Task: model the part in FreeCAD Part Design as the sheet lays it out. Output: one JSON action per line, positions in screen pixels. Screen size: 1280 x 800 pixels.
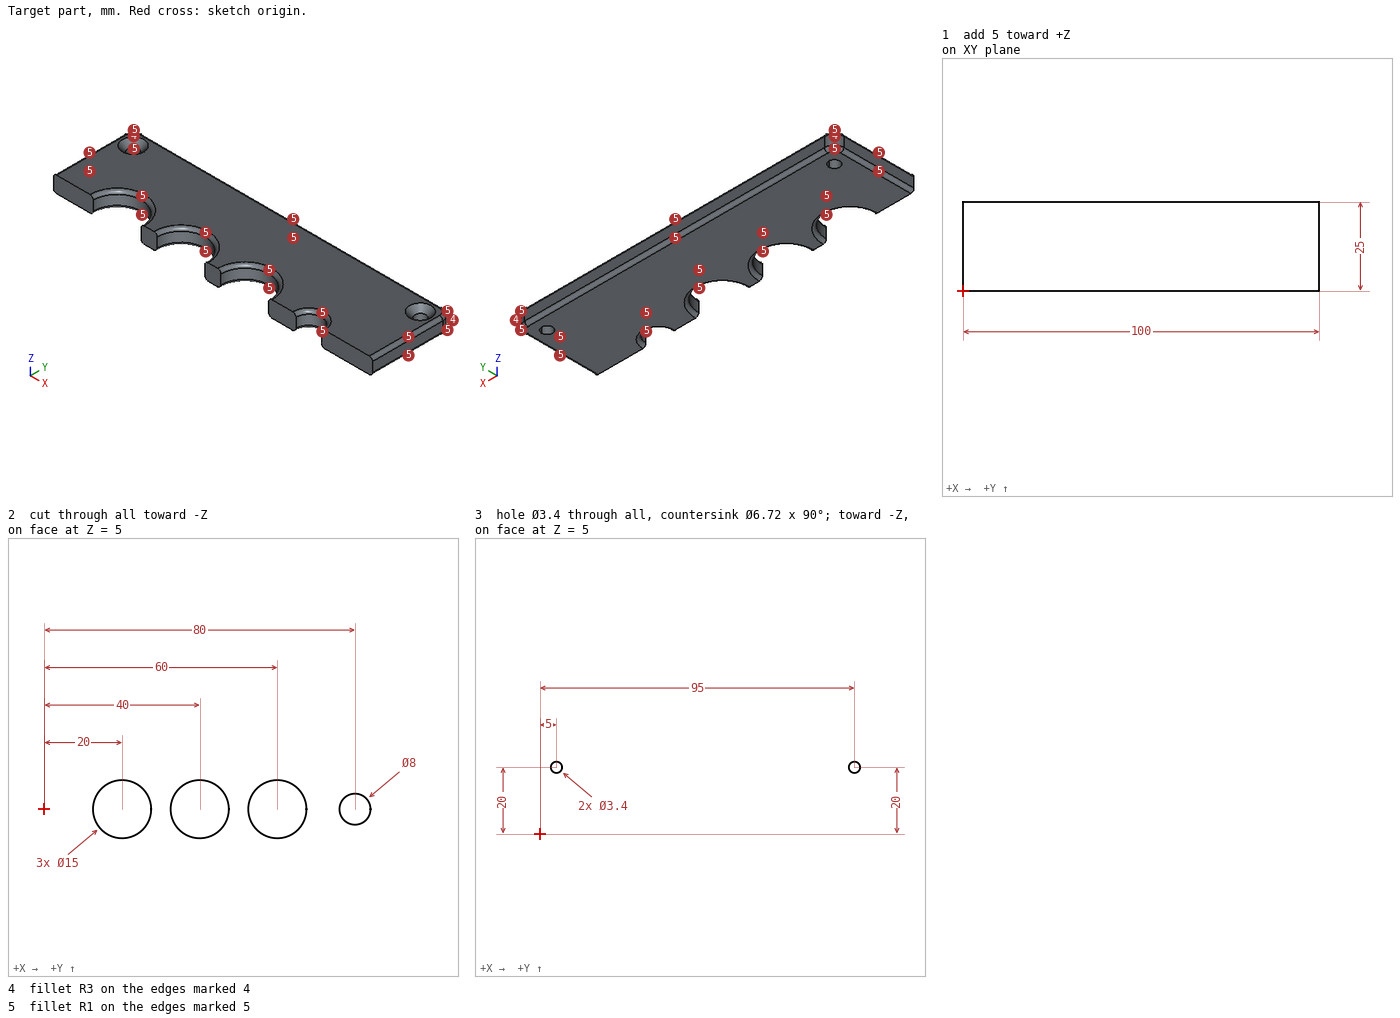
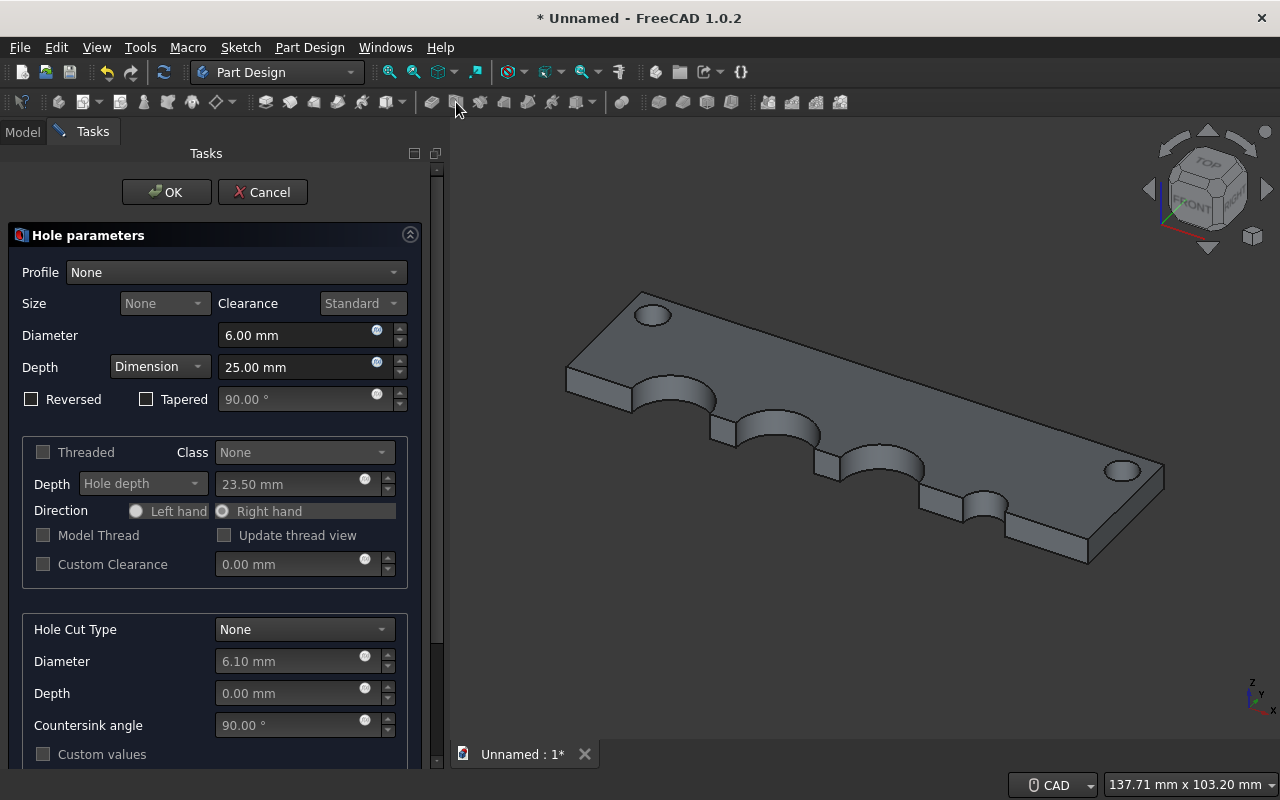
{"action": "triple_click", "coordinate": [305, 335]}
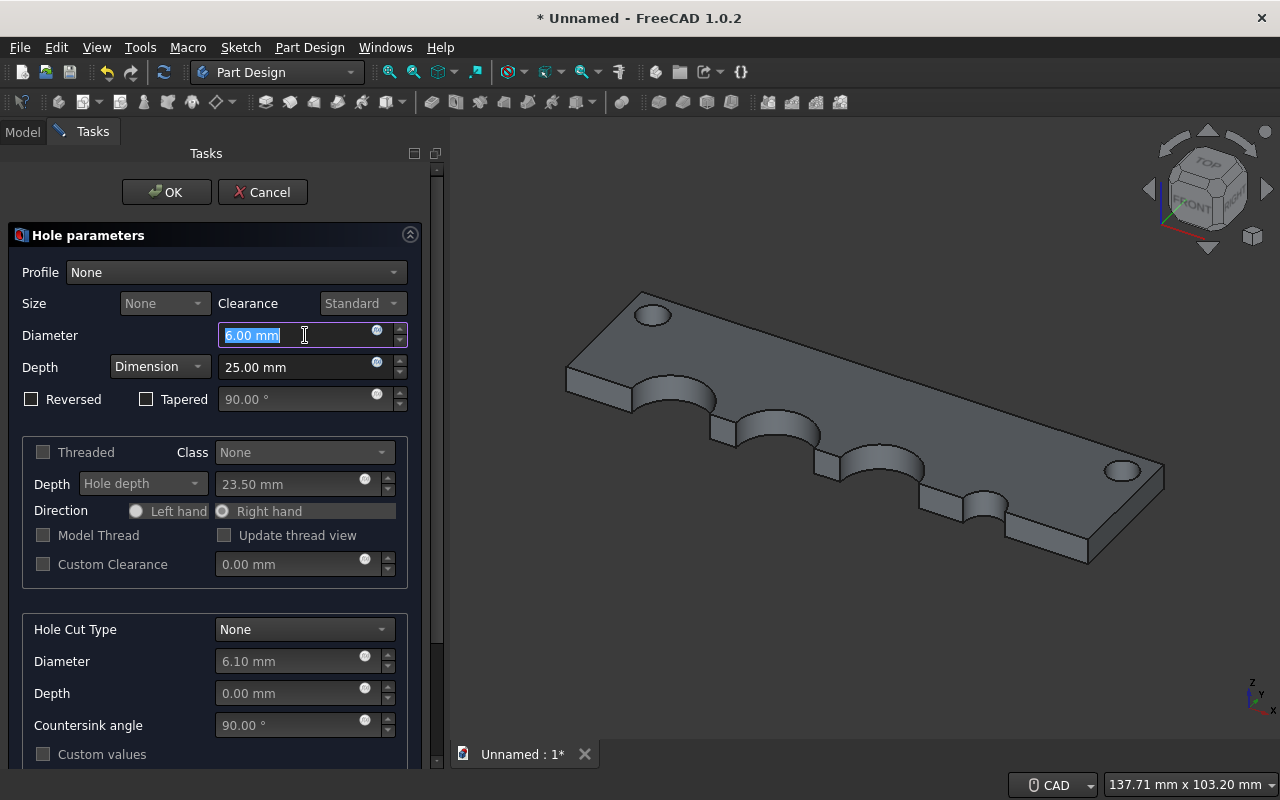
{"action": "type", "text": "3.4"}
{"action": "key", "text": "Tab"}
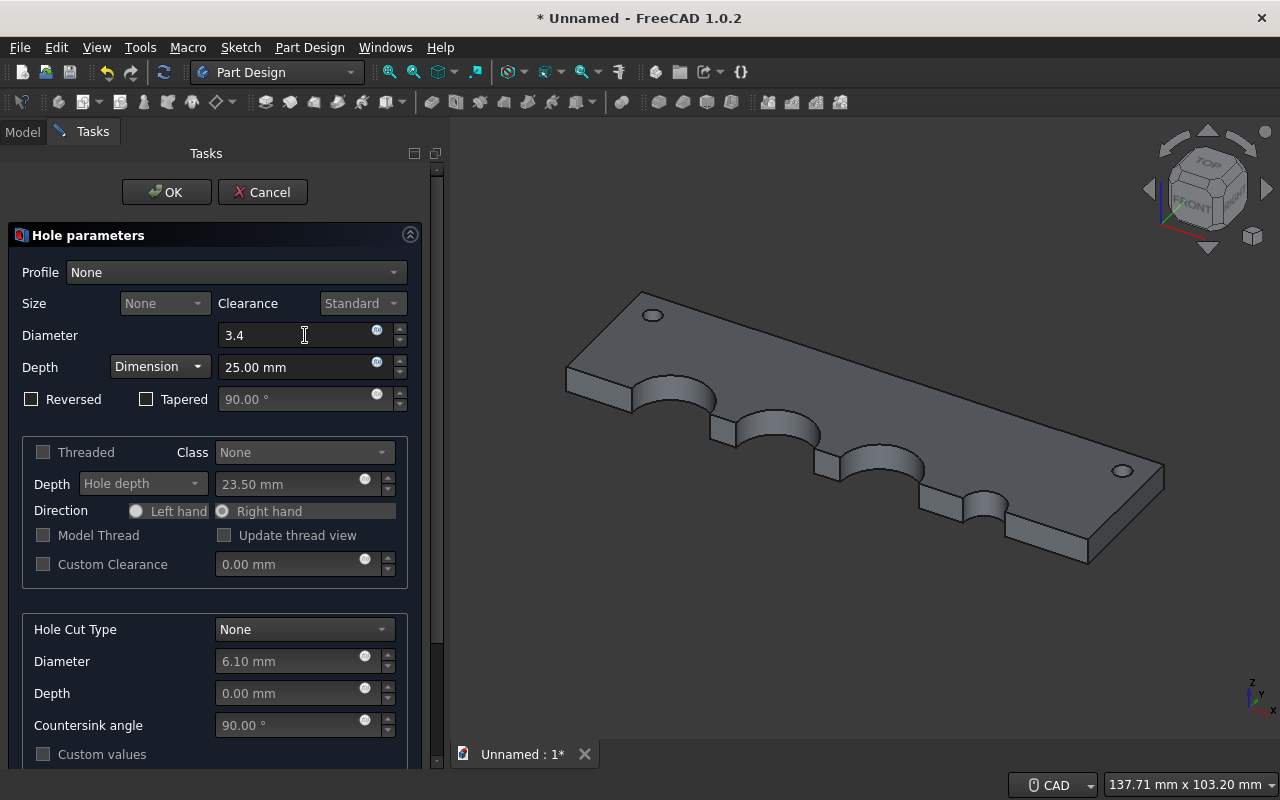
{"action": "left_click", "coordinate": [161, 366]}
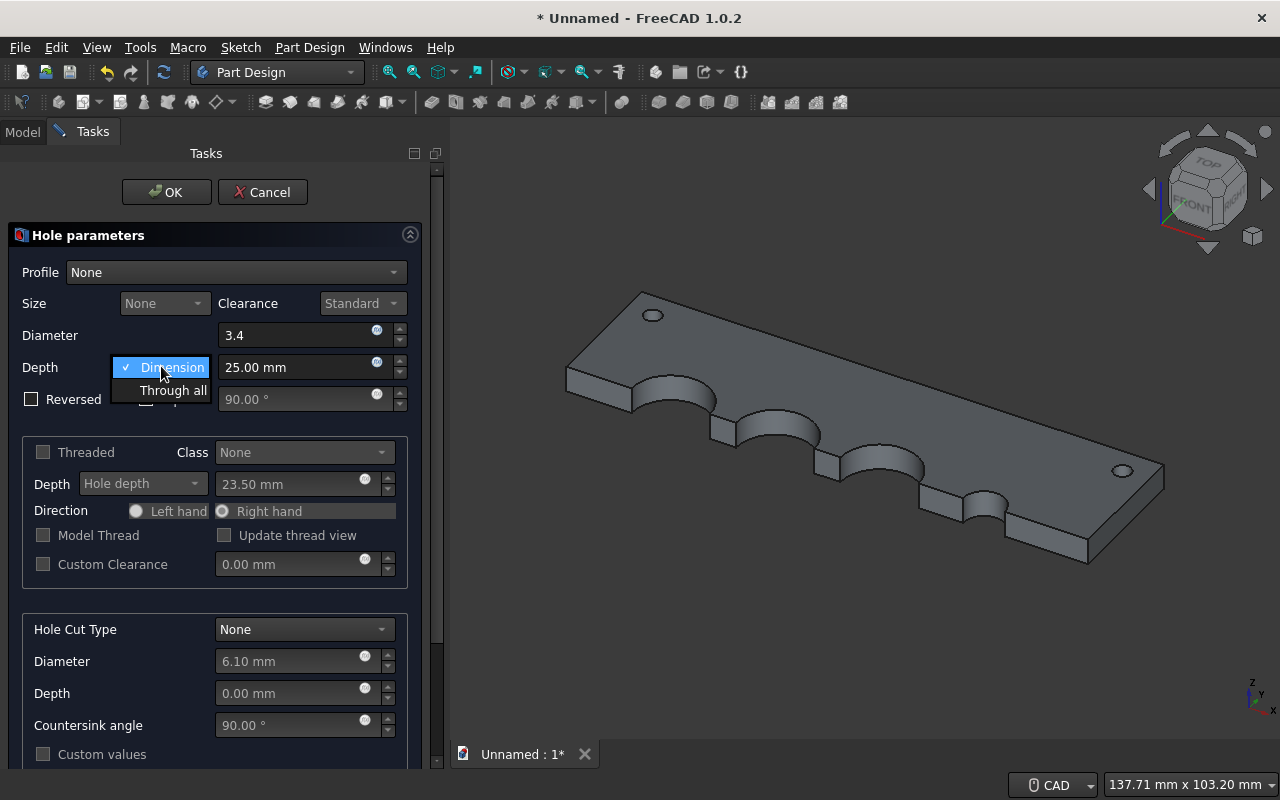
{"action": "left_click", "coordinate": [160, 390]}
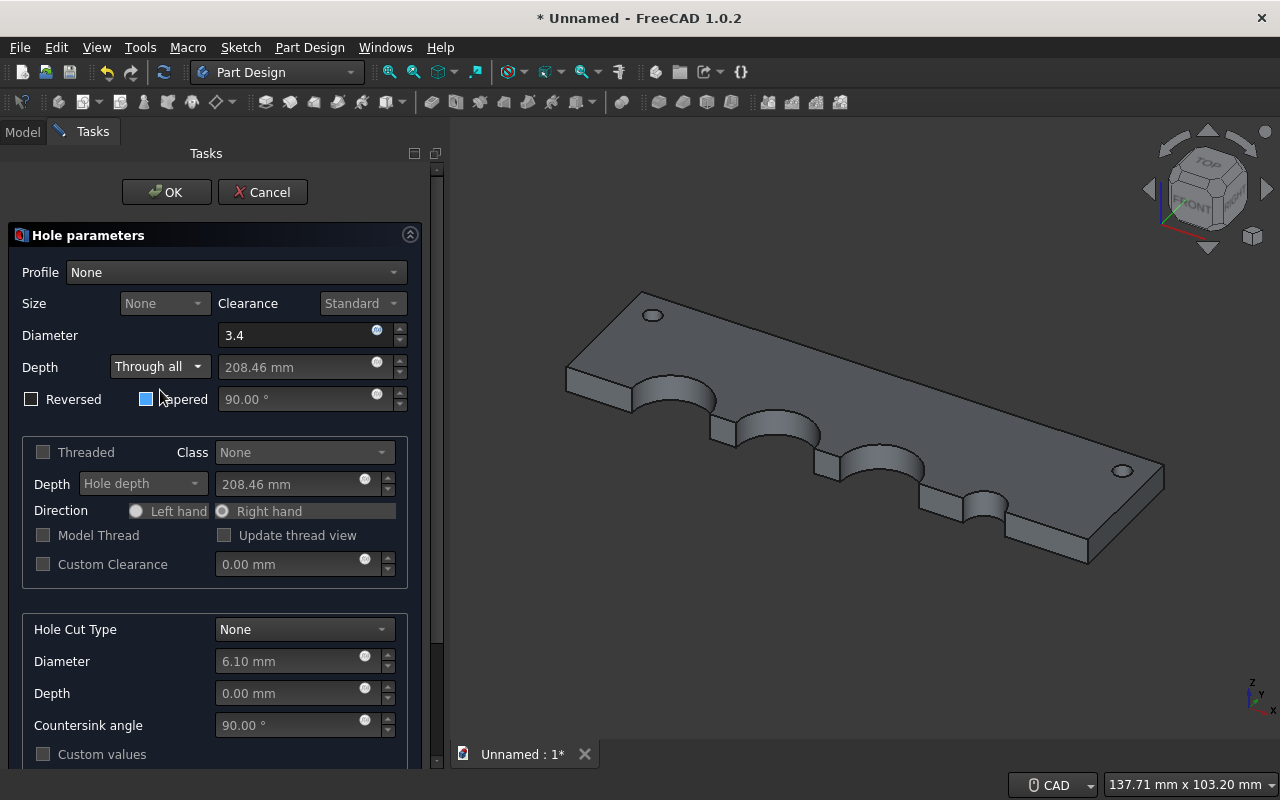
{"action": "left_click", "coordinate": [306, 630]}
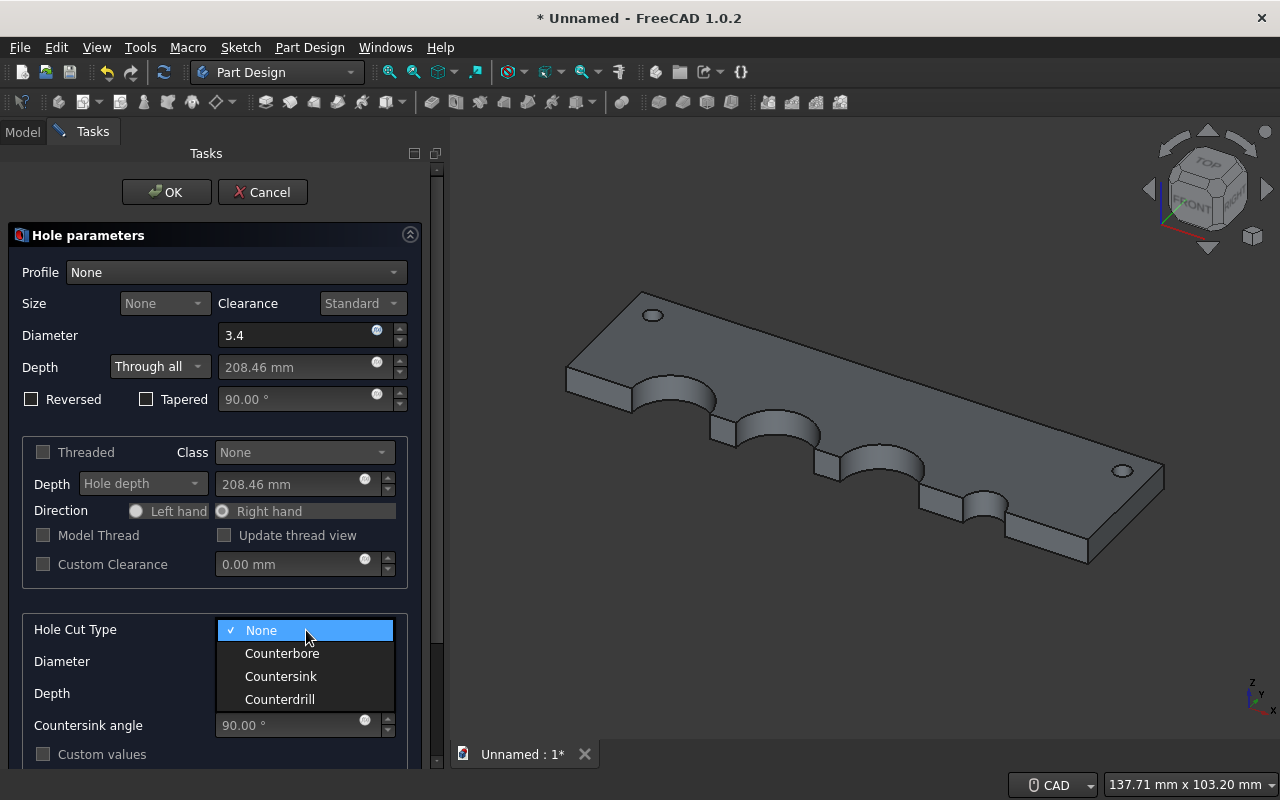
{"action": "left_click", "coordinate": [304, 676]}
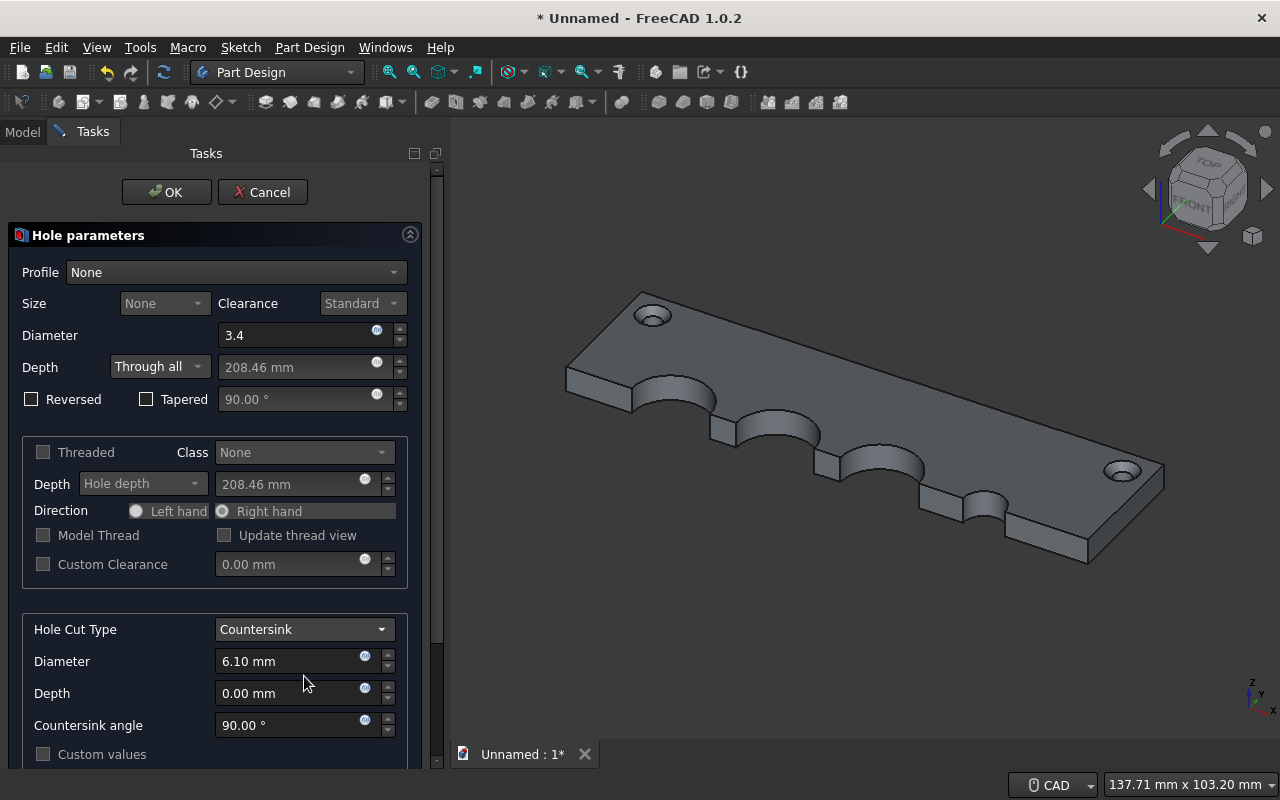
{"action": "triple_click", "coordinate": [298, 661]}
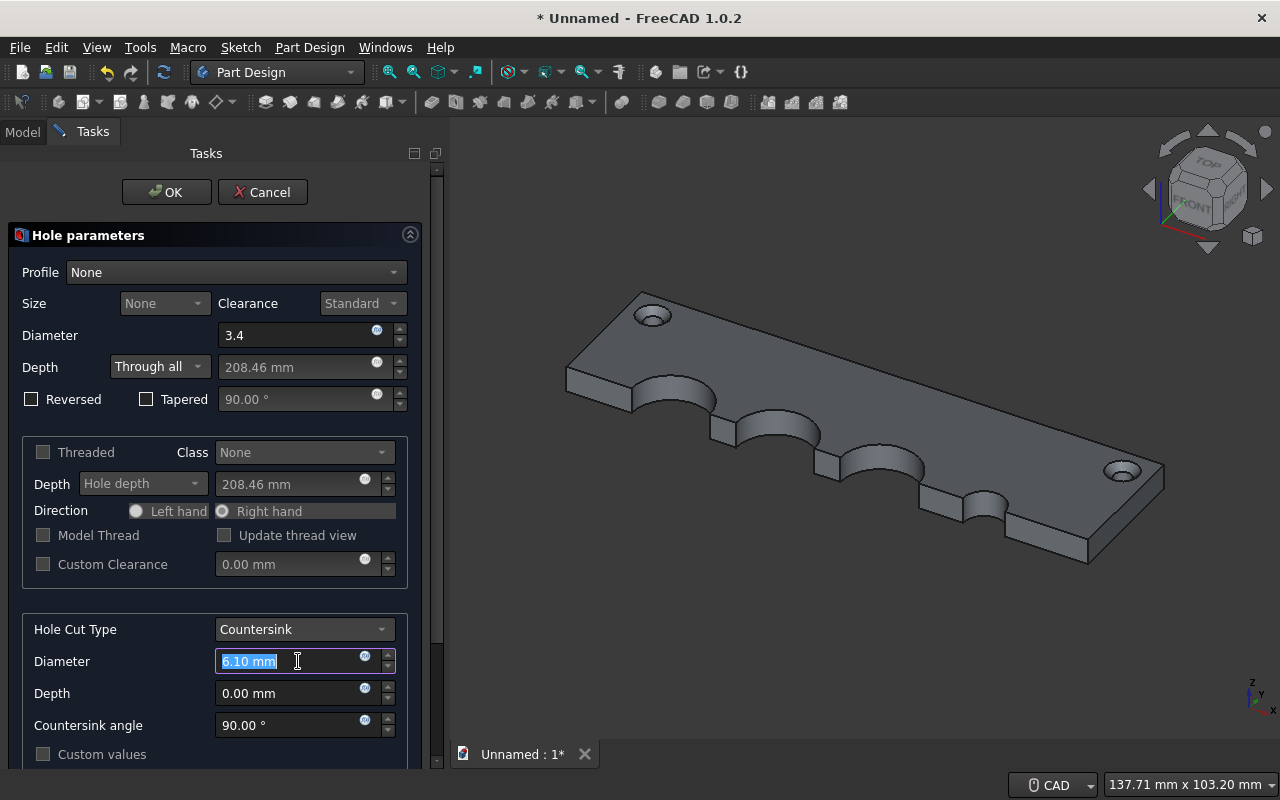
{"action": "type", "text": "6.72"}
{"action": "key", "text": "Tab"}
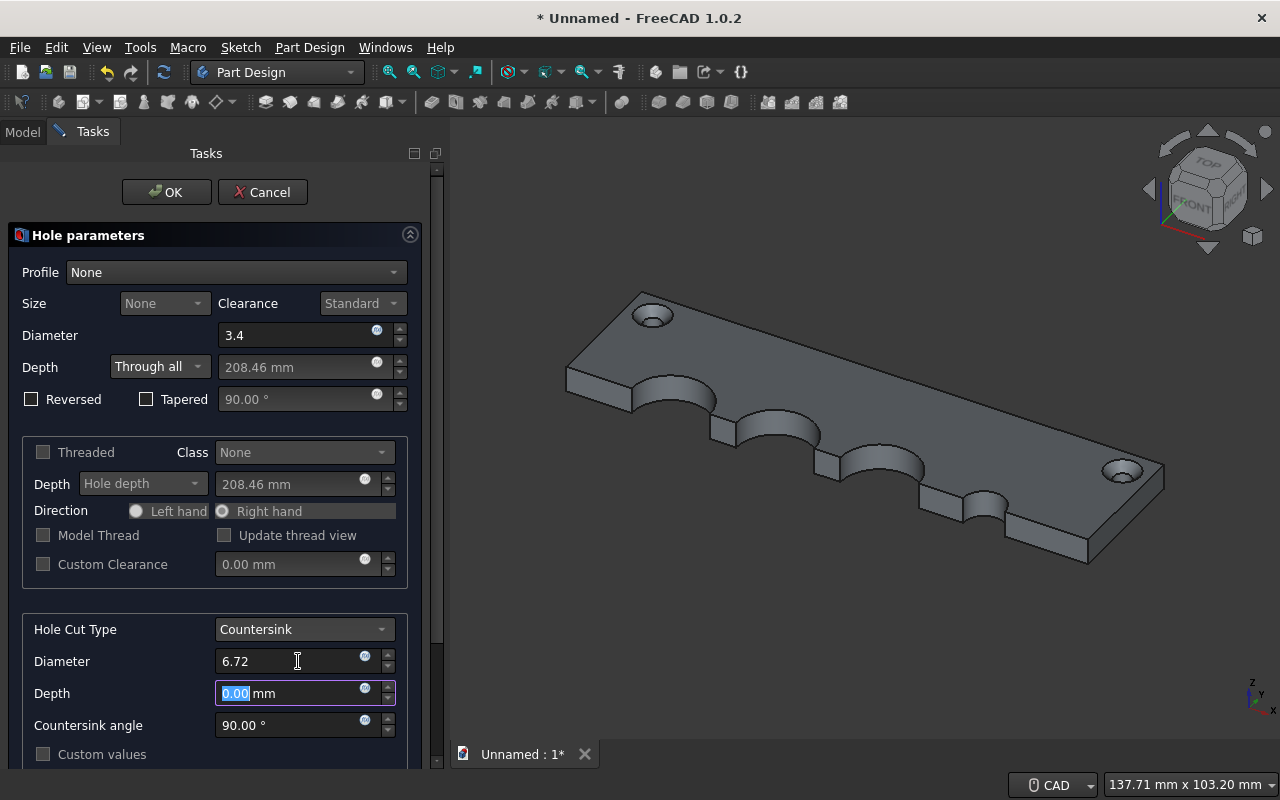
{"action": "left_click", "coordinate": [167, 192]}